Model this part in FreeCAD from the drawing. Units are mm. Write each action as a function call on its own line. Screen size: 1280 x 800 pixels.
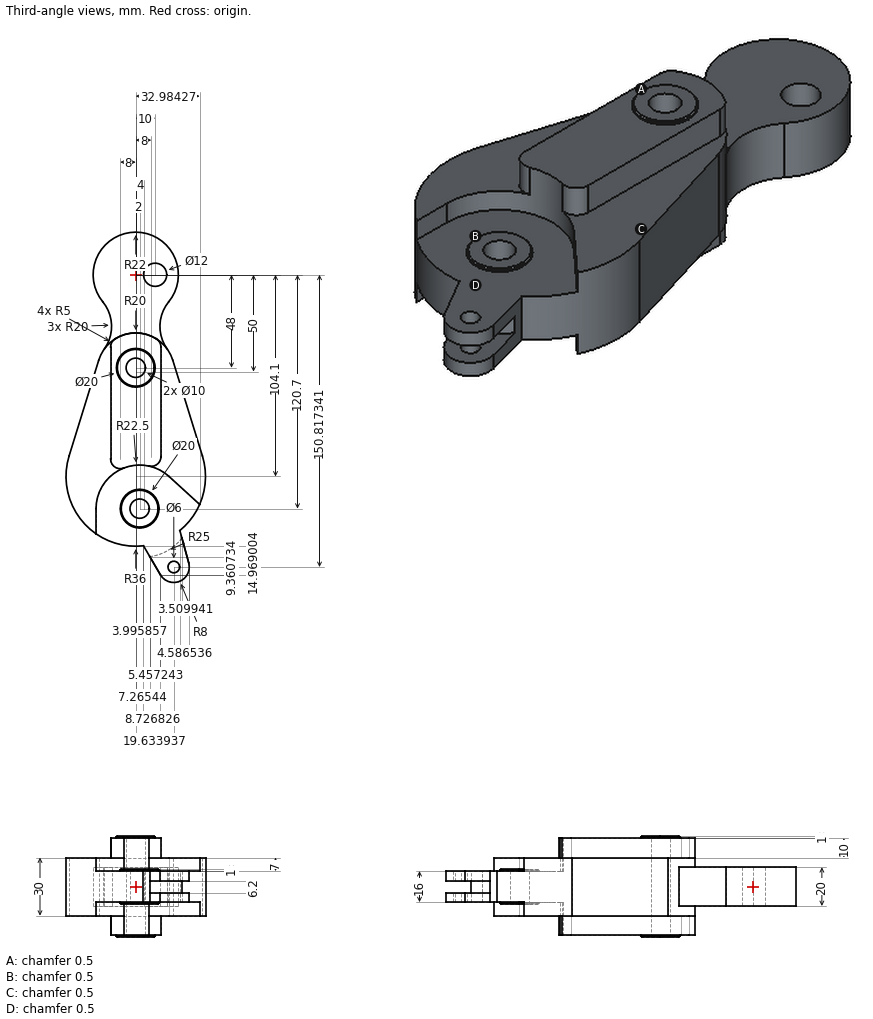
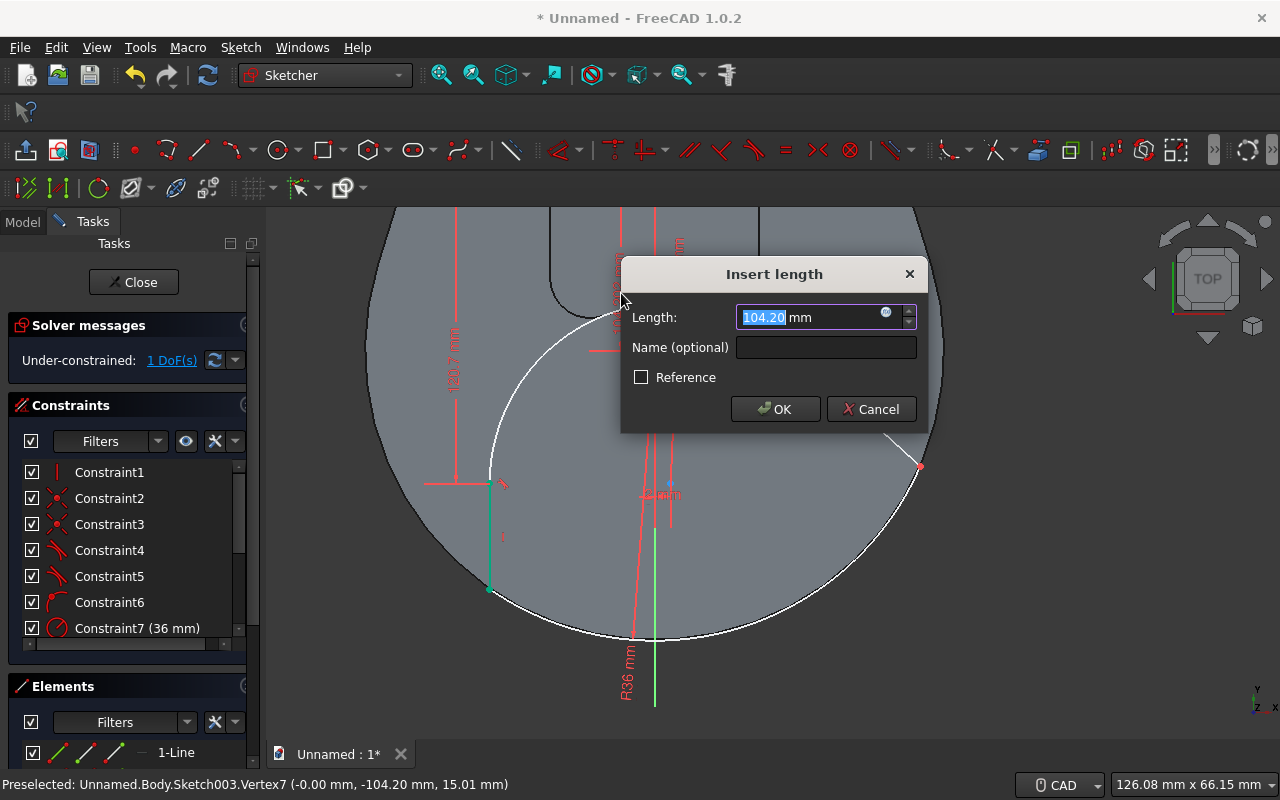
text(104.1)
key(Return)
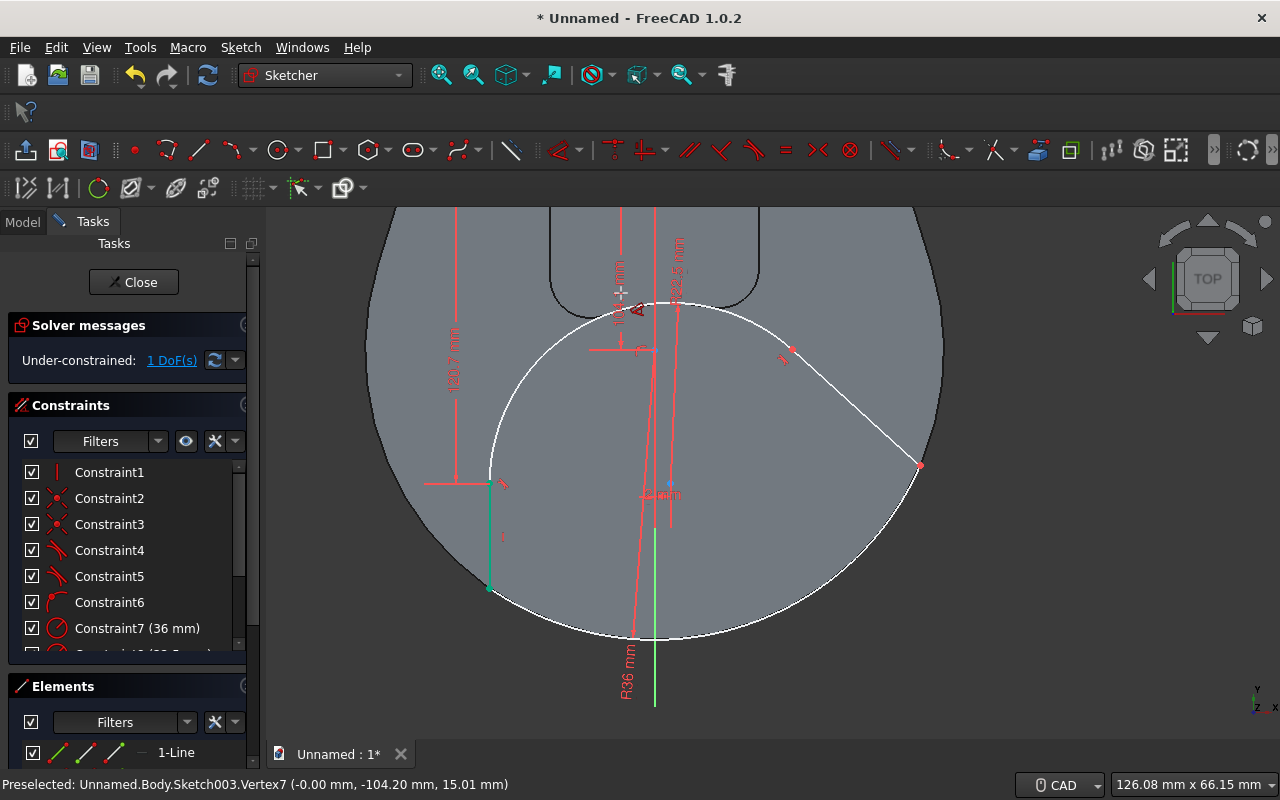
click(920, 466)
click(787, 500)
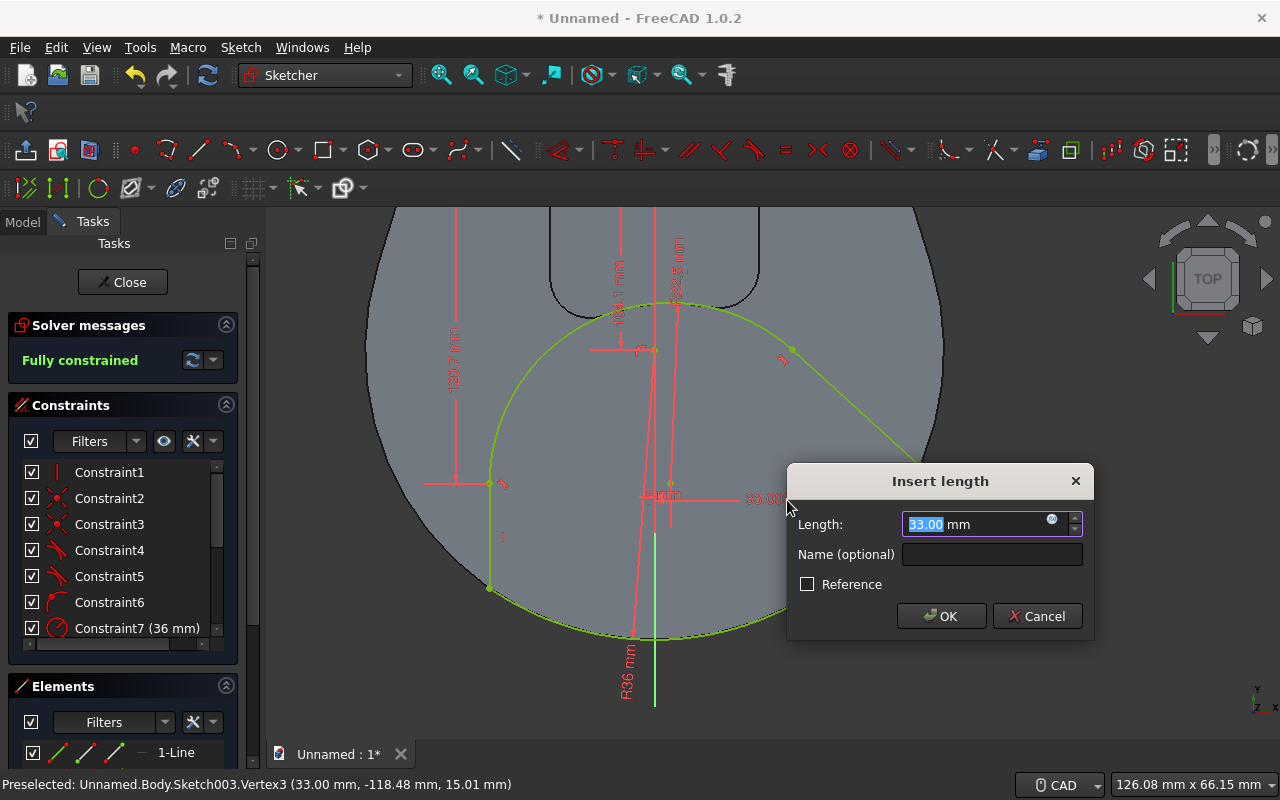
text(32.98427)
key(Return)
key(Escape)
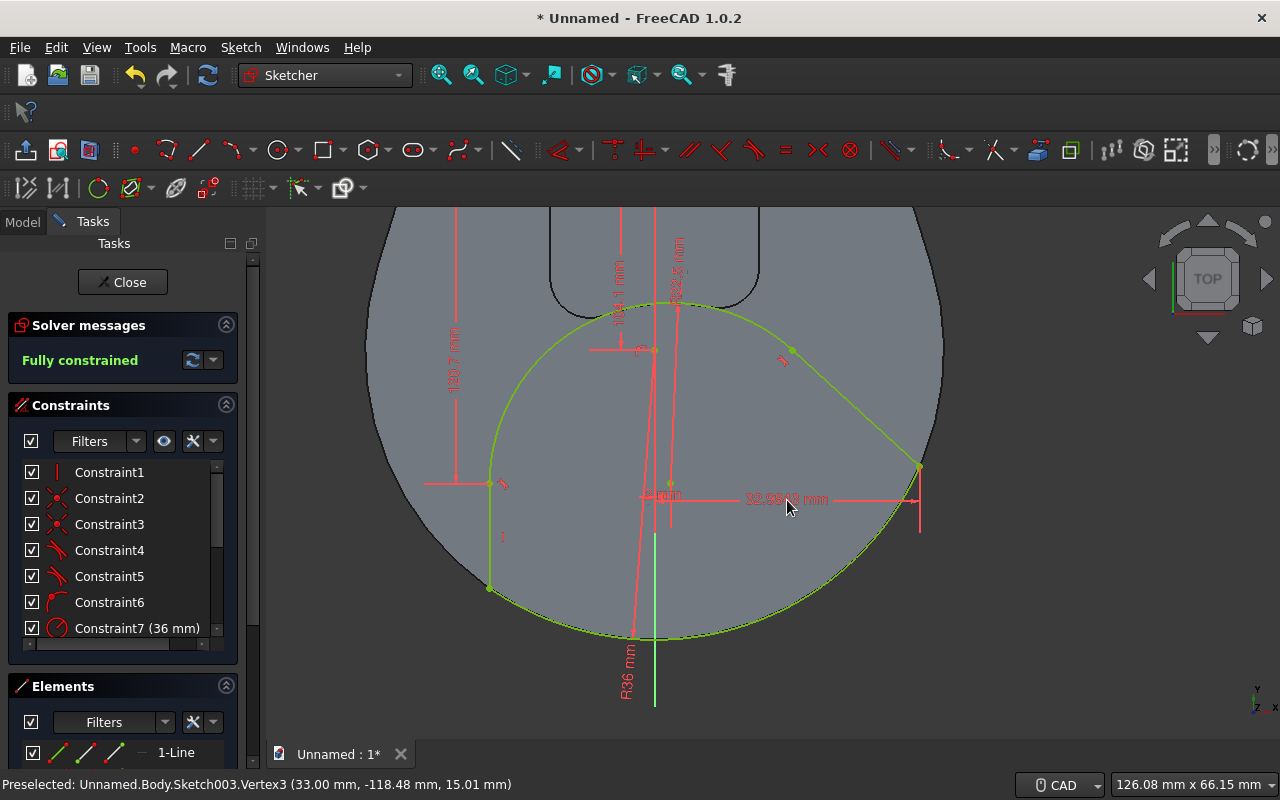
click(123, 282)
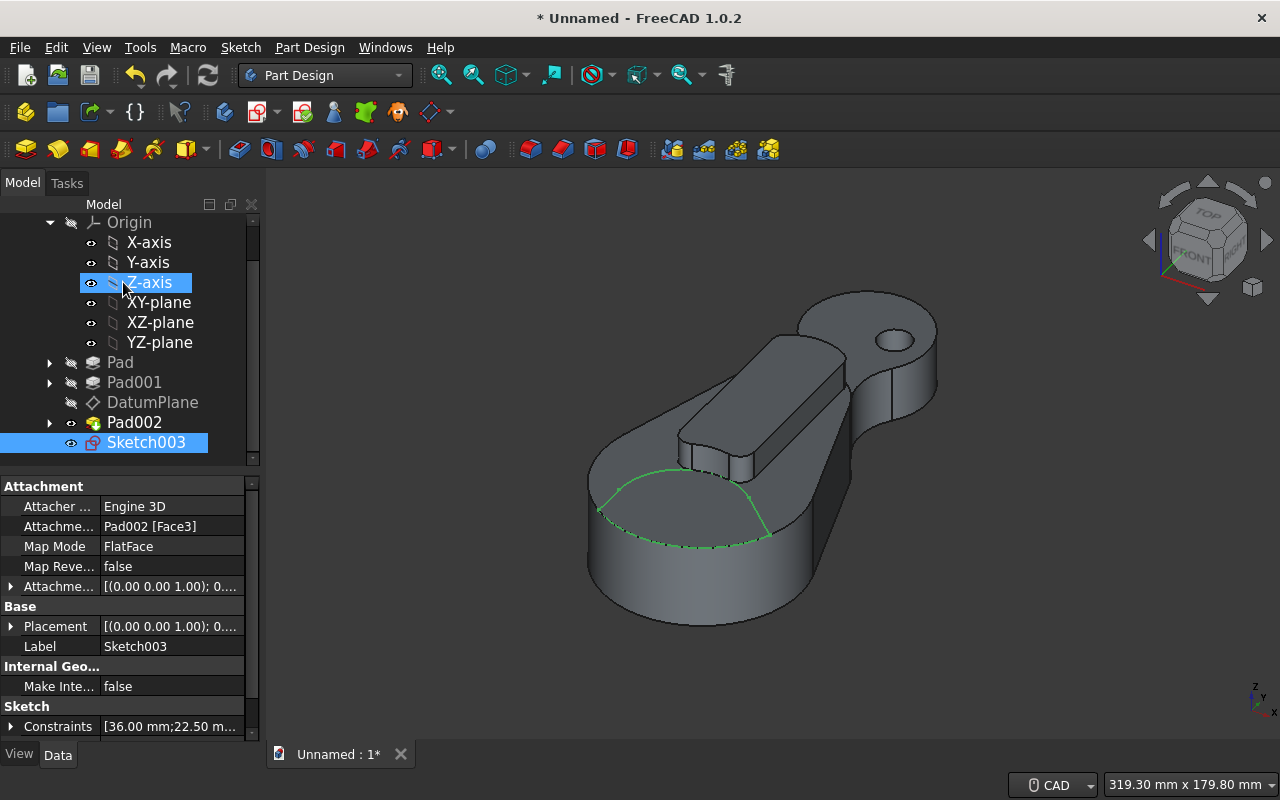
click(240, 150)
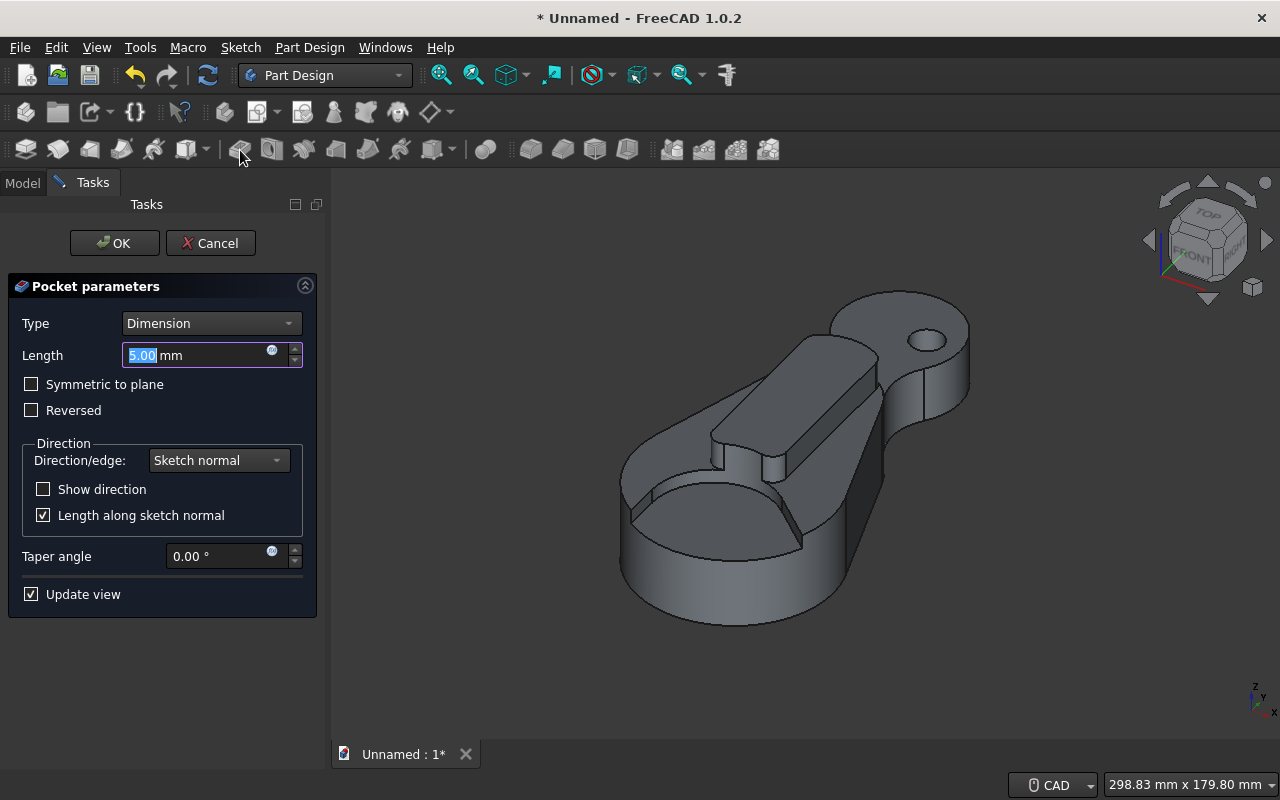
text(7)
key(Tab)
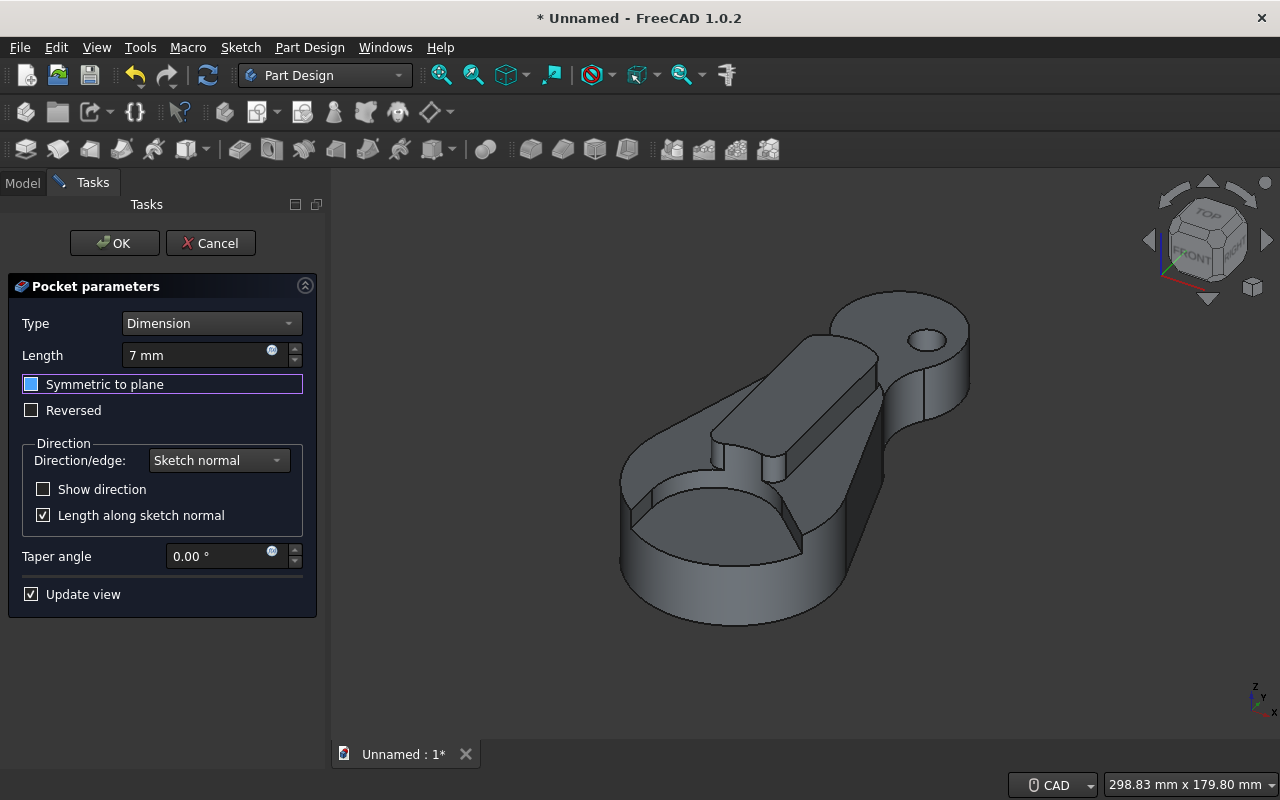
click(115, 243)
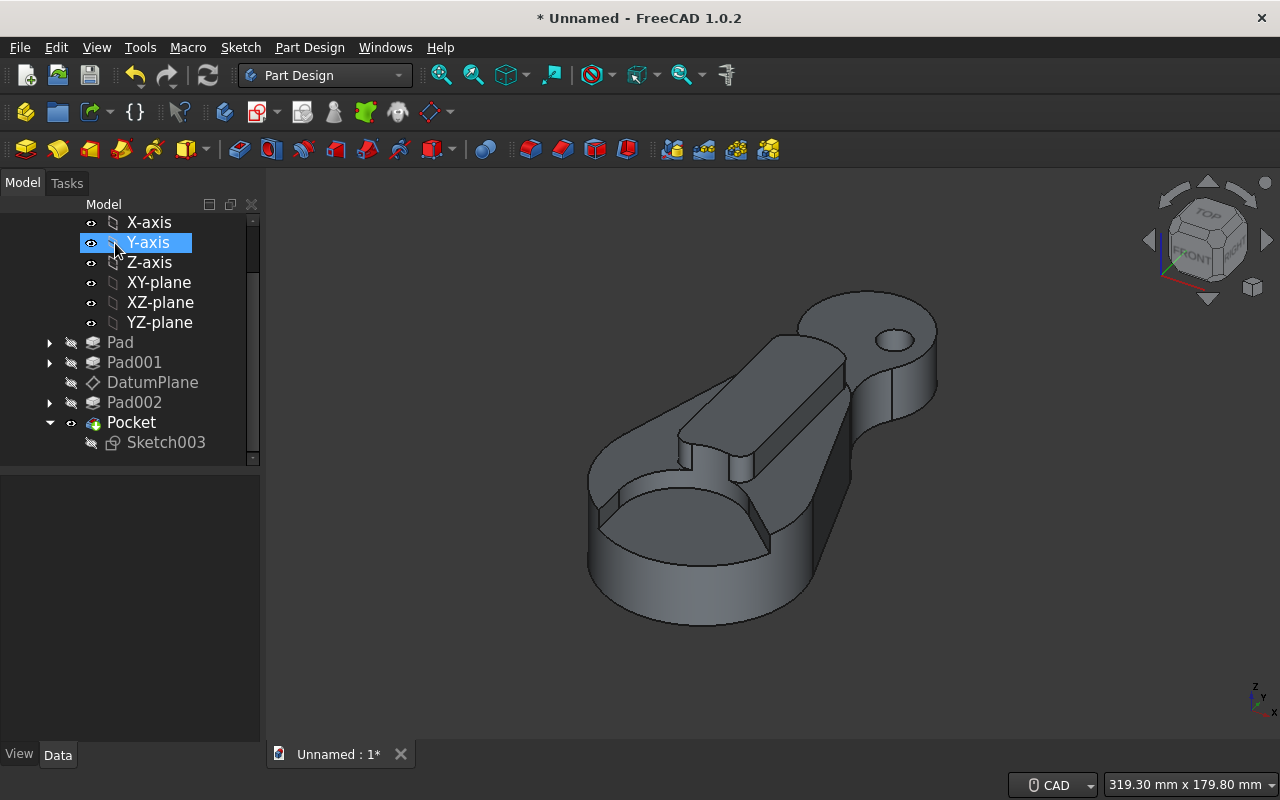
click(116, 403)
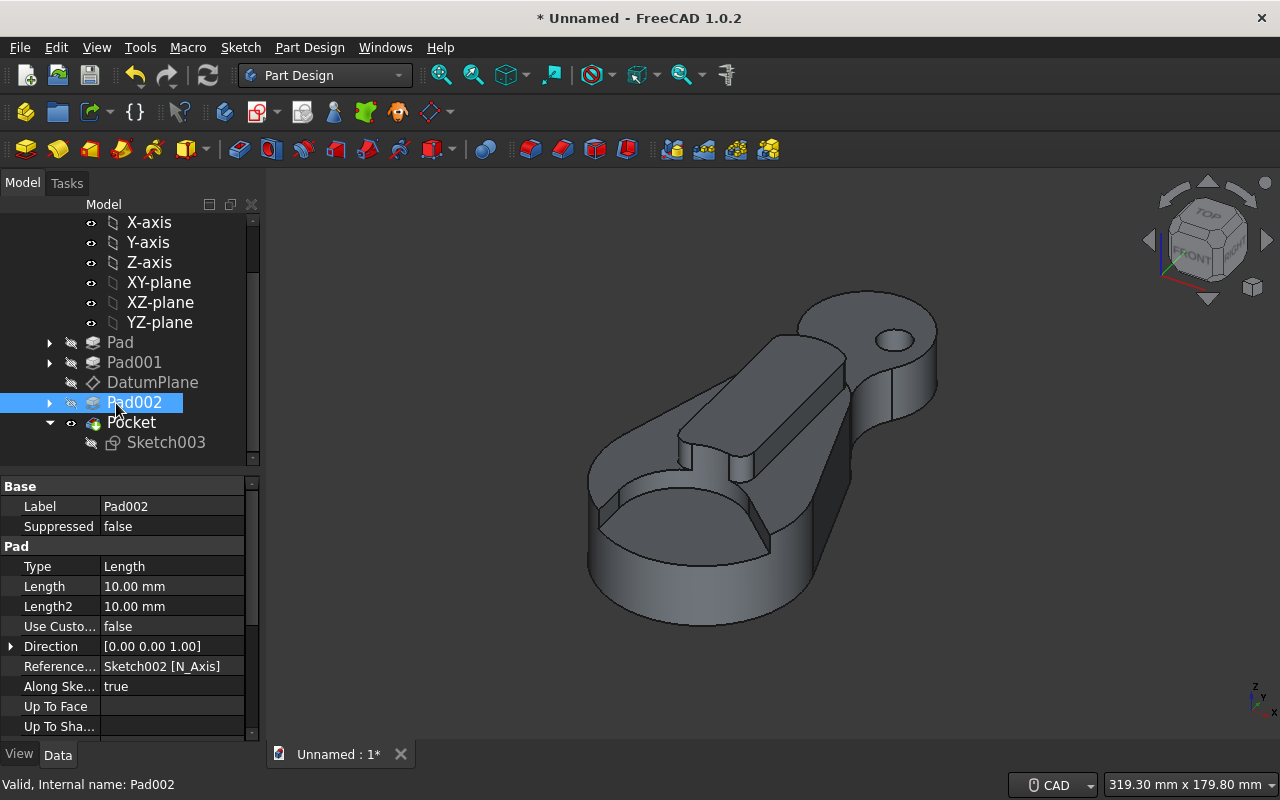
click(116, 423, ctrl)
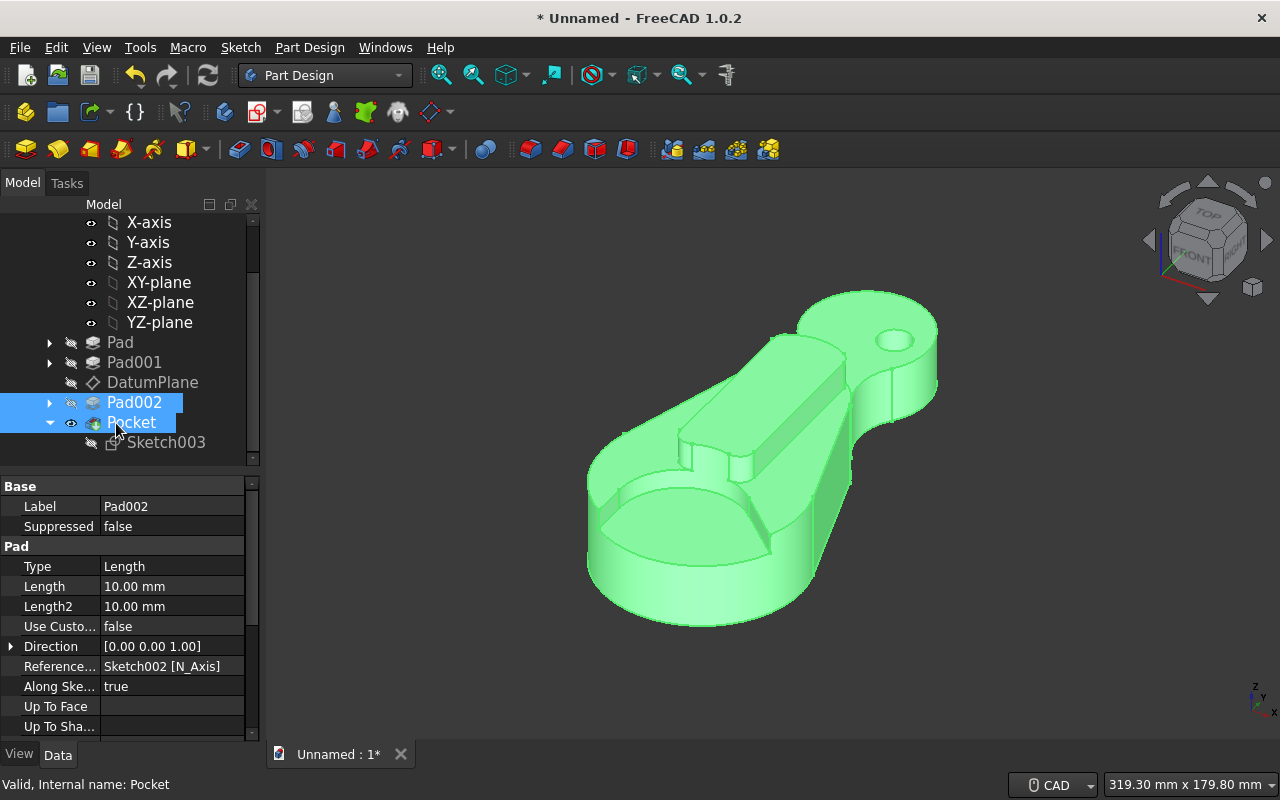
click(672, 150)